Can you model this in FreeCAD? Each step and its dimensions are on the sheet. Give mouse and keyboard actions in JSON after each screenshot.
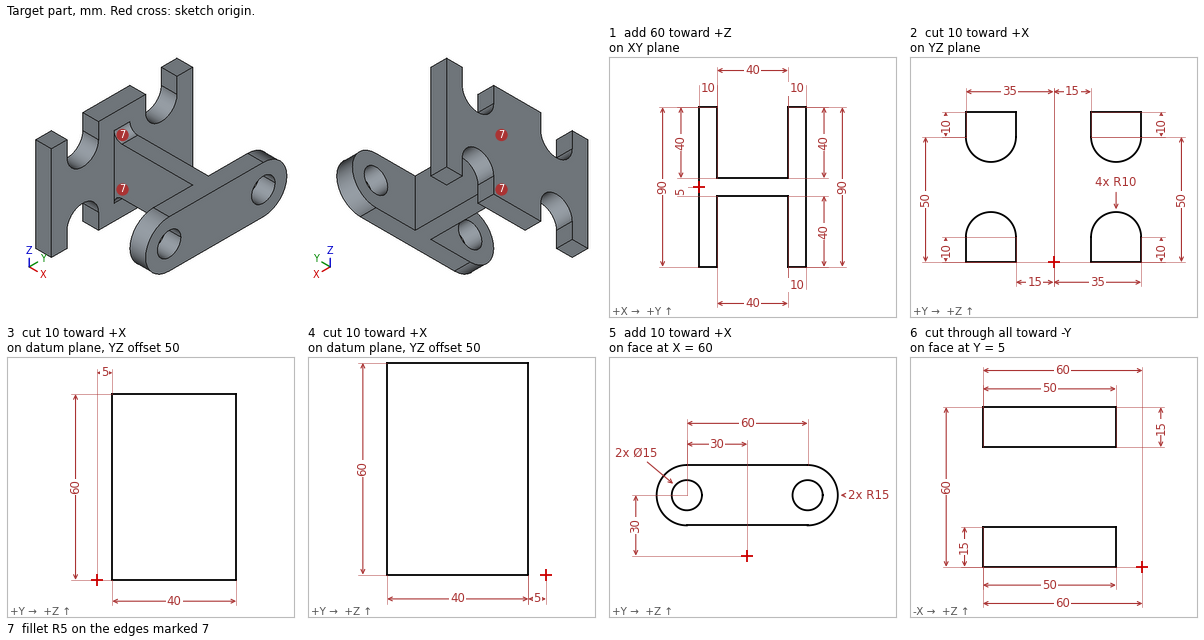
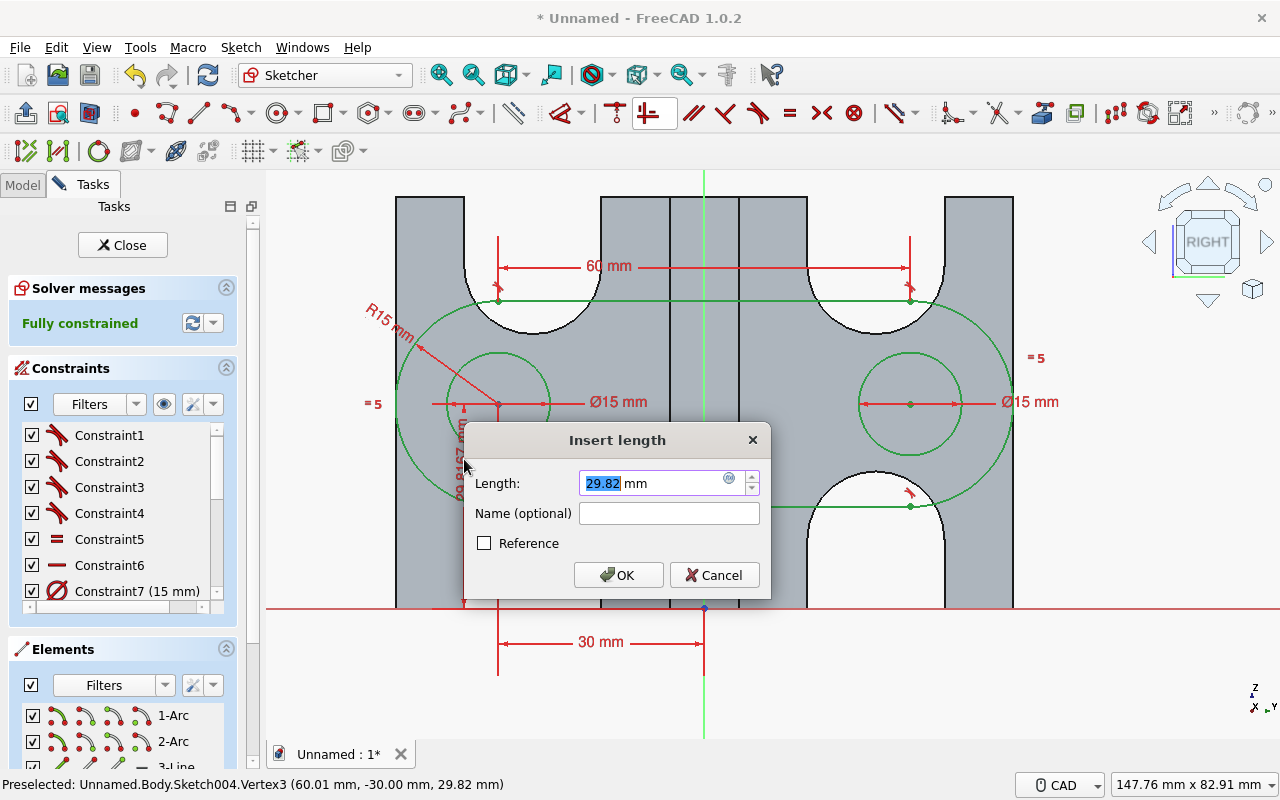
{"action": "type", "text": "30"}
{"action": "key", "text": "Return"}
{"action": "key", "text": "Escape"}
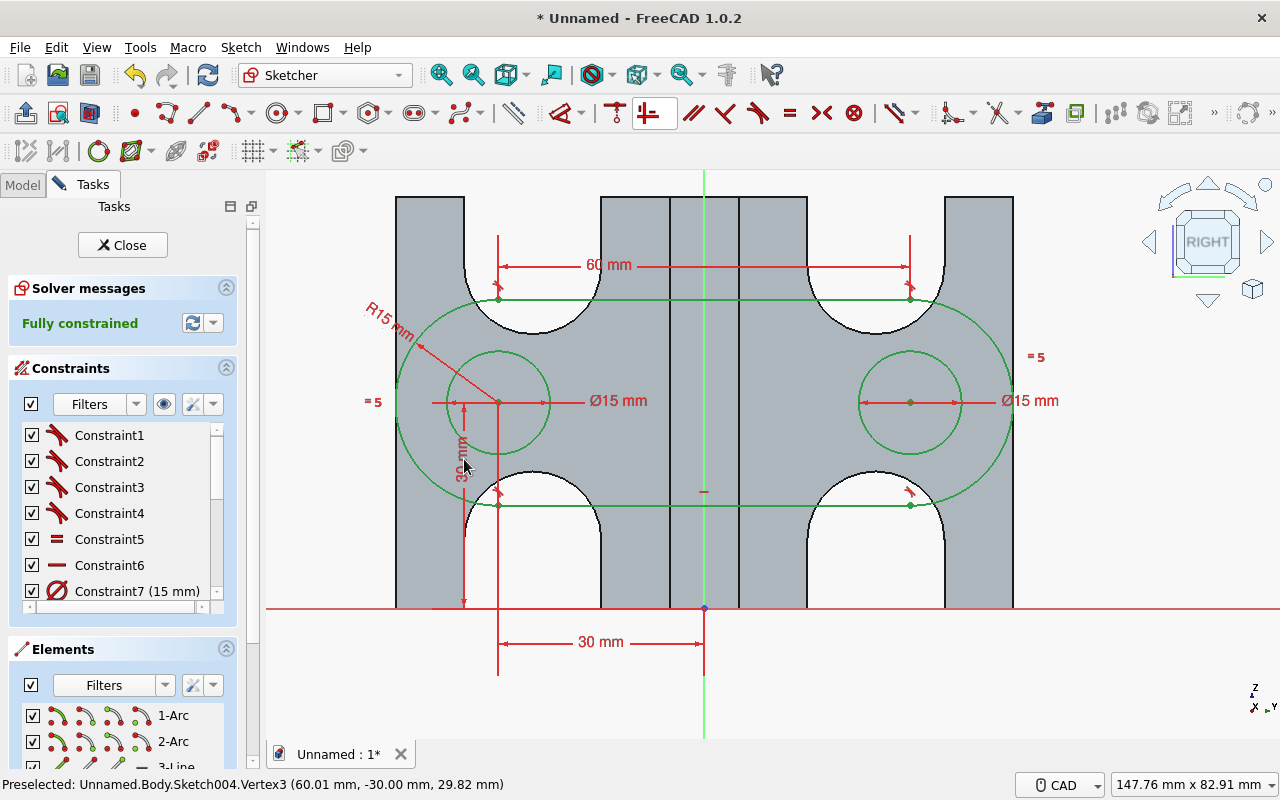
{"action": "left_click", "coordinate": [123, 245]}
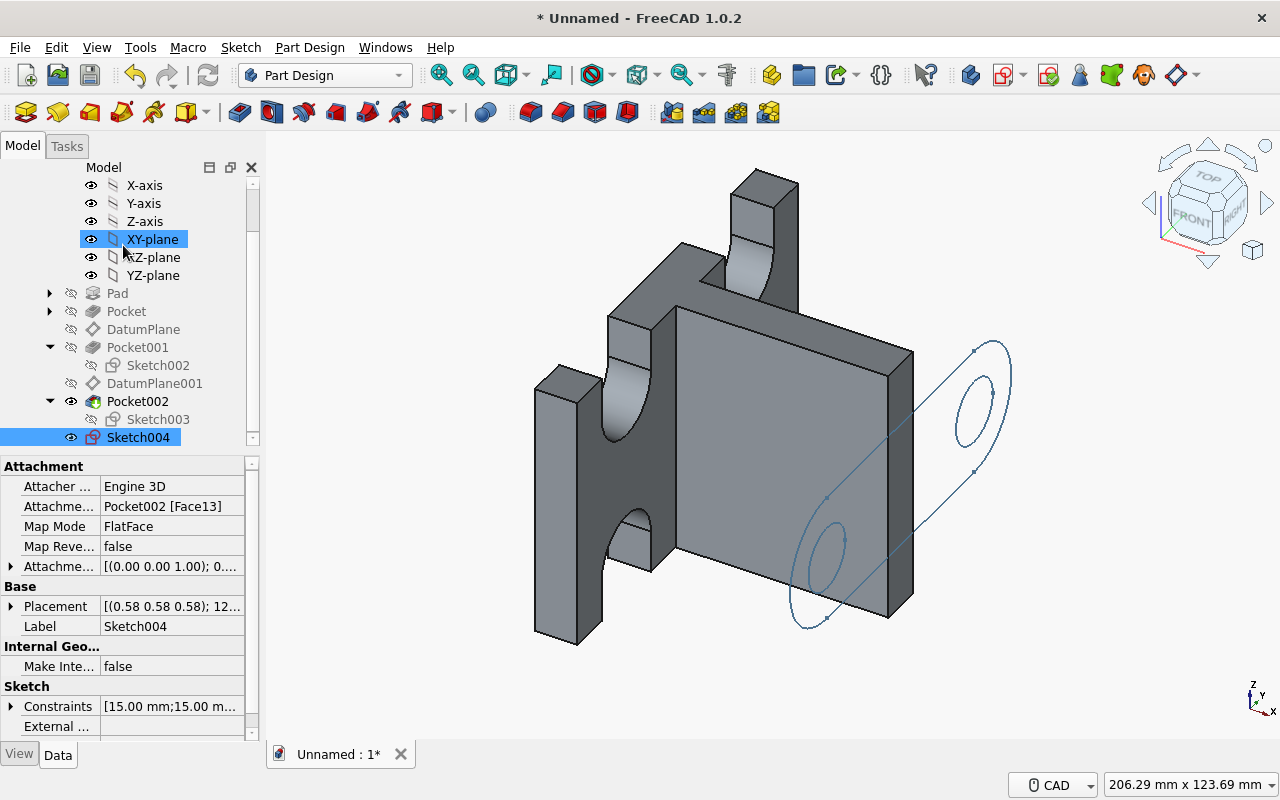
{"action": "left_click", "coordinate": [26, 112]}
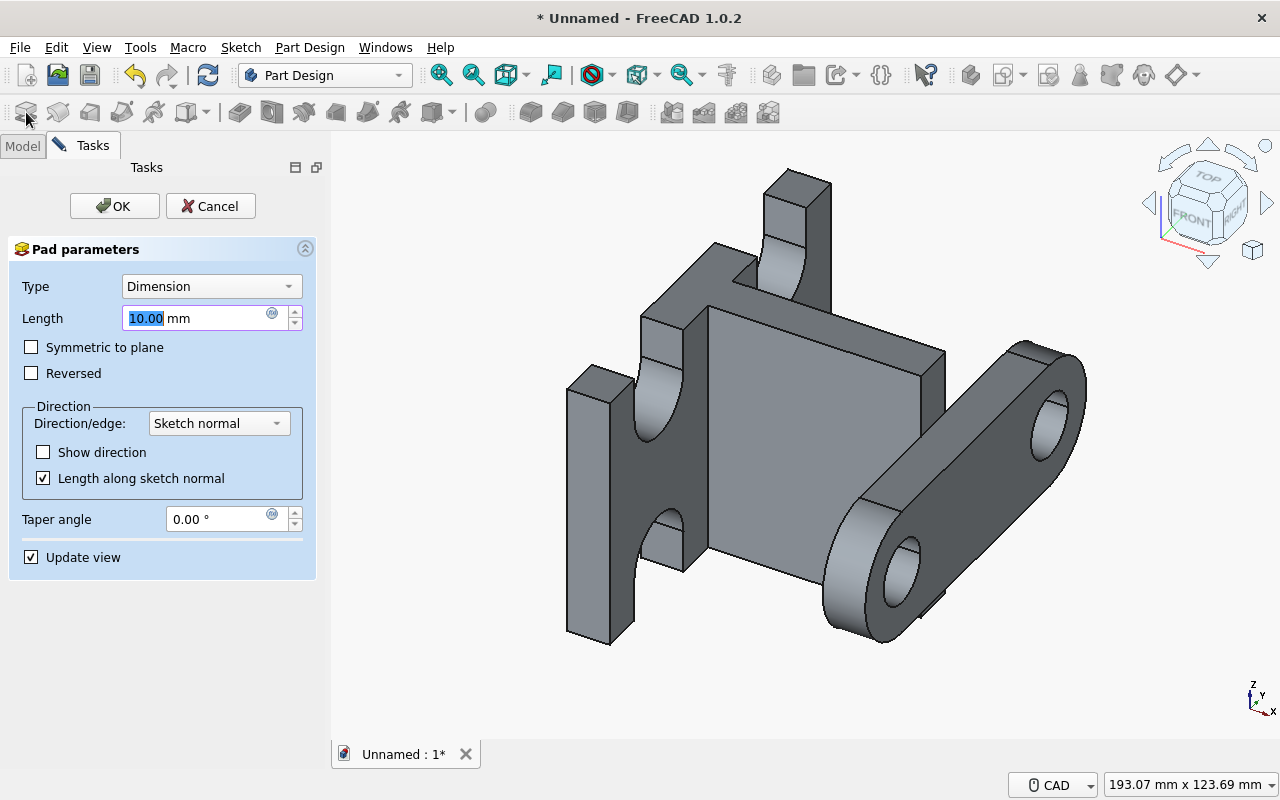
{"action": "type", "text": "10"}
{"action": "key", "text": "Tab"}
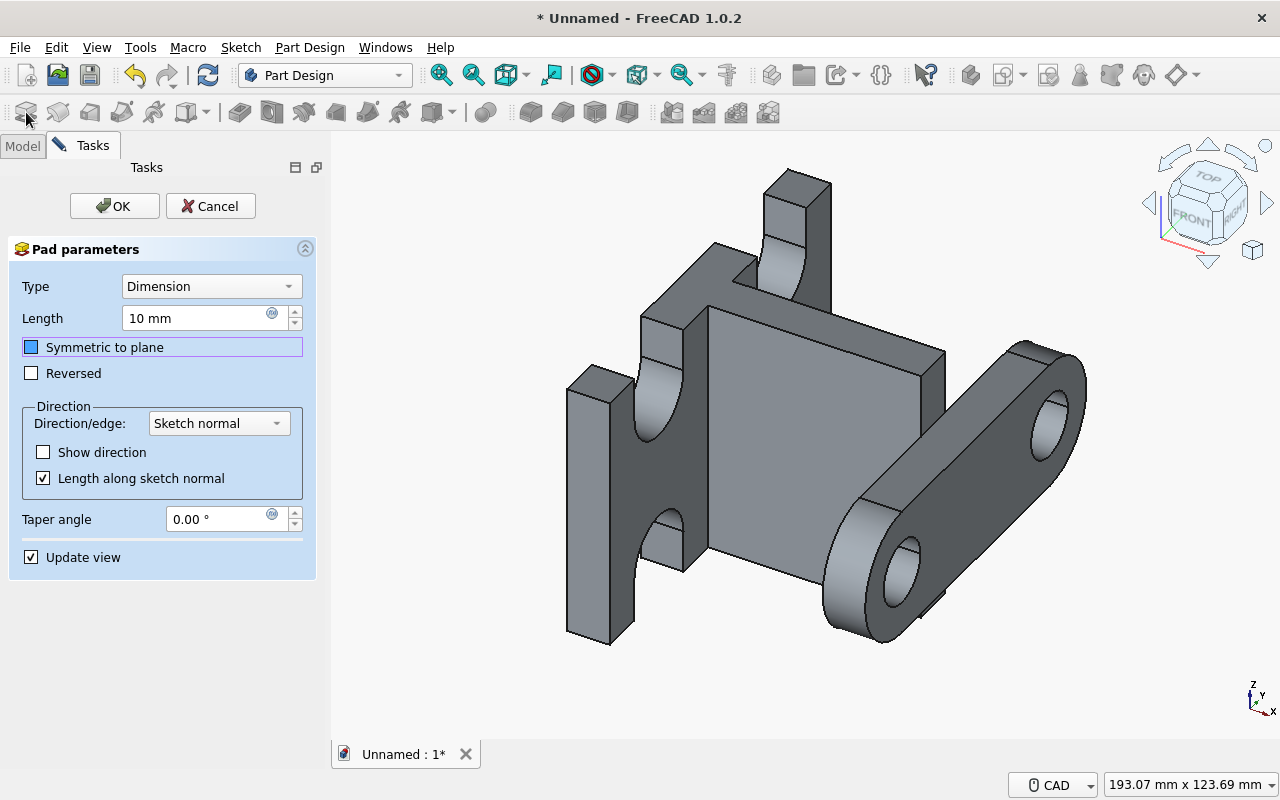
{"action": "left_click", "coordinate": [115, 206]}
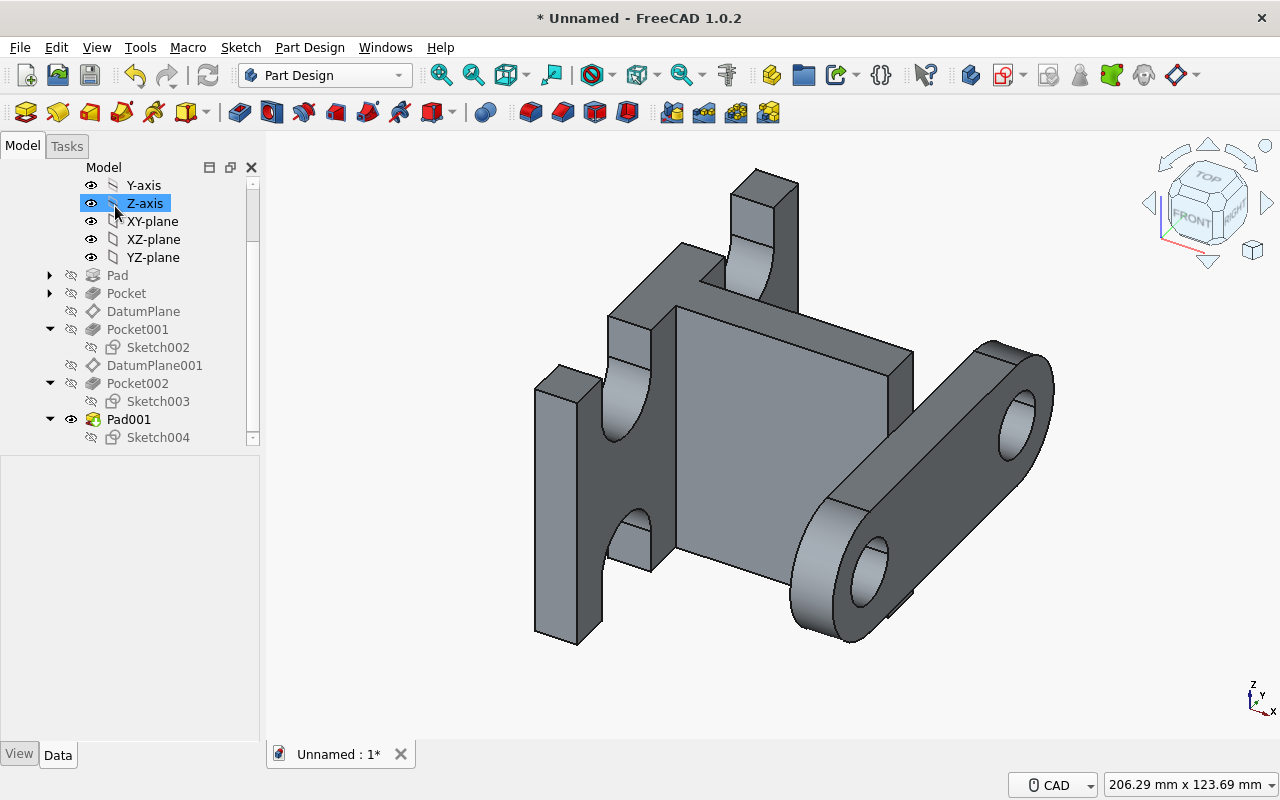
{"action": "key", "text": "4"}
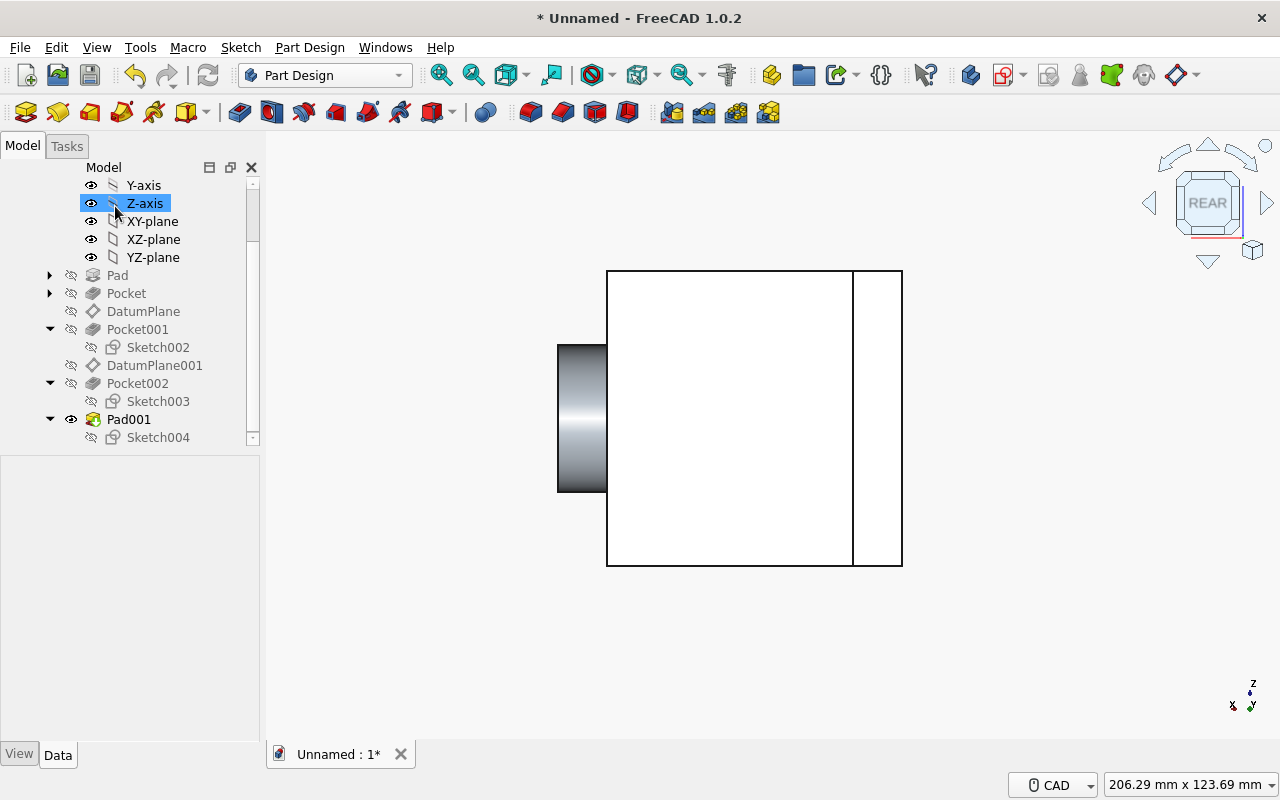
{"action": "left_click", "coordinate": [730, 417]}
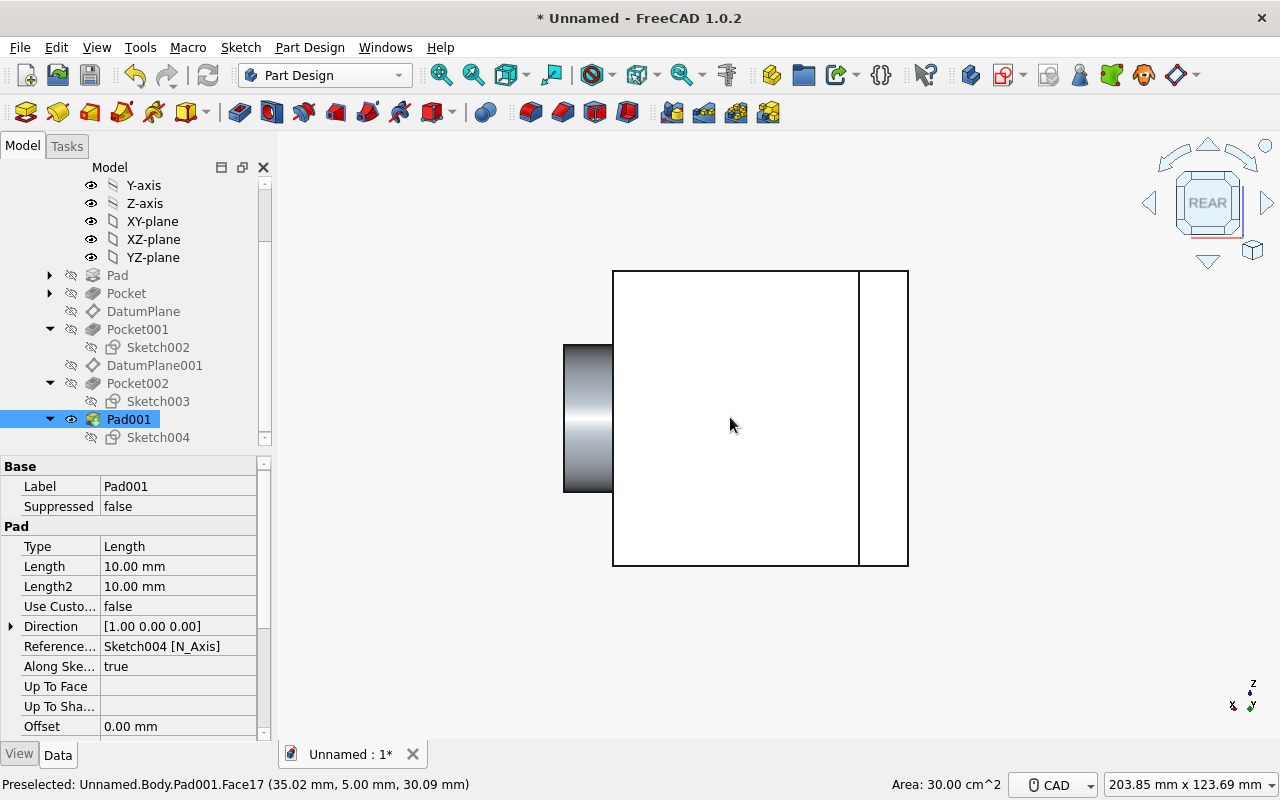
{"action": "left_click", "coordinate": [1004, 76]}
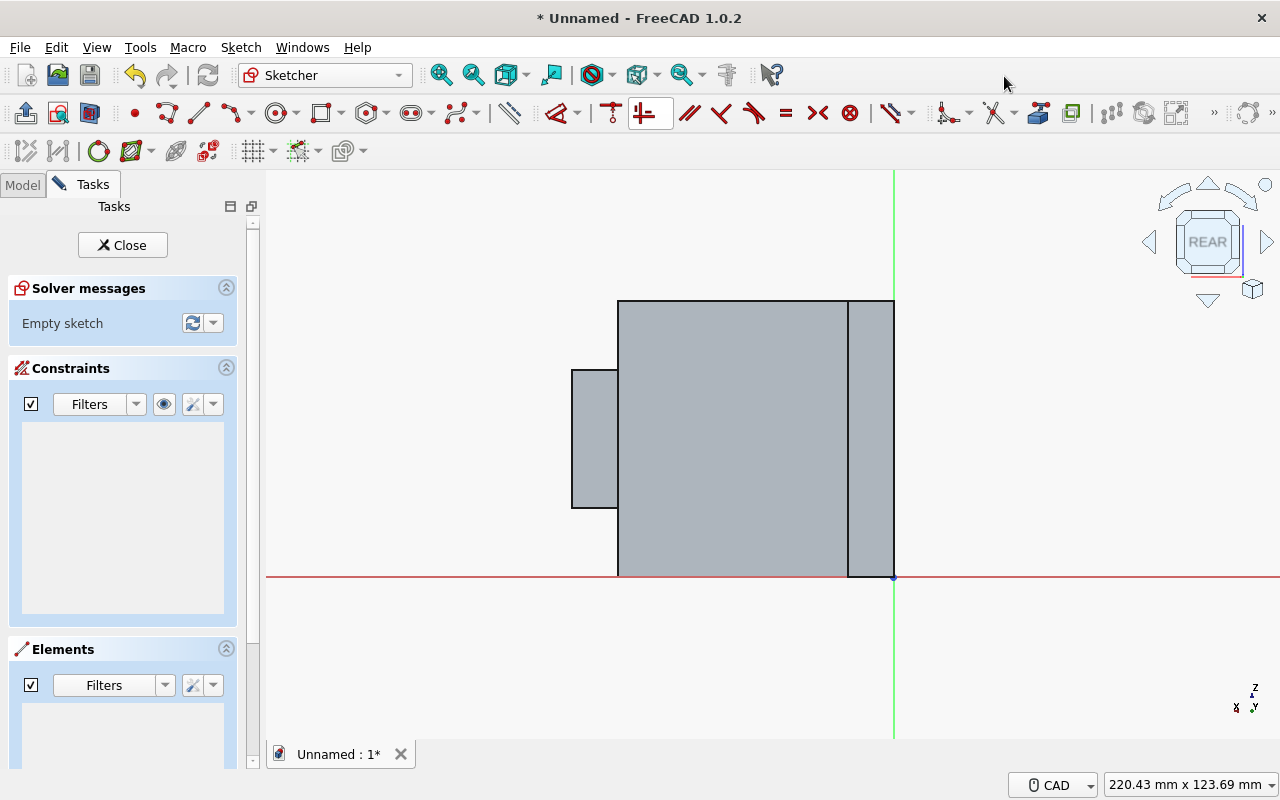
{"action": "left_click", "coordinate": [90, 114]}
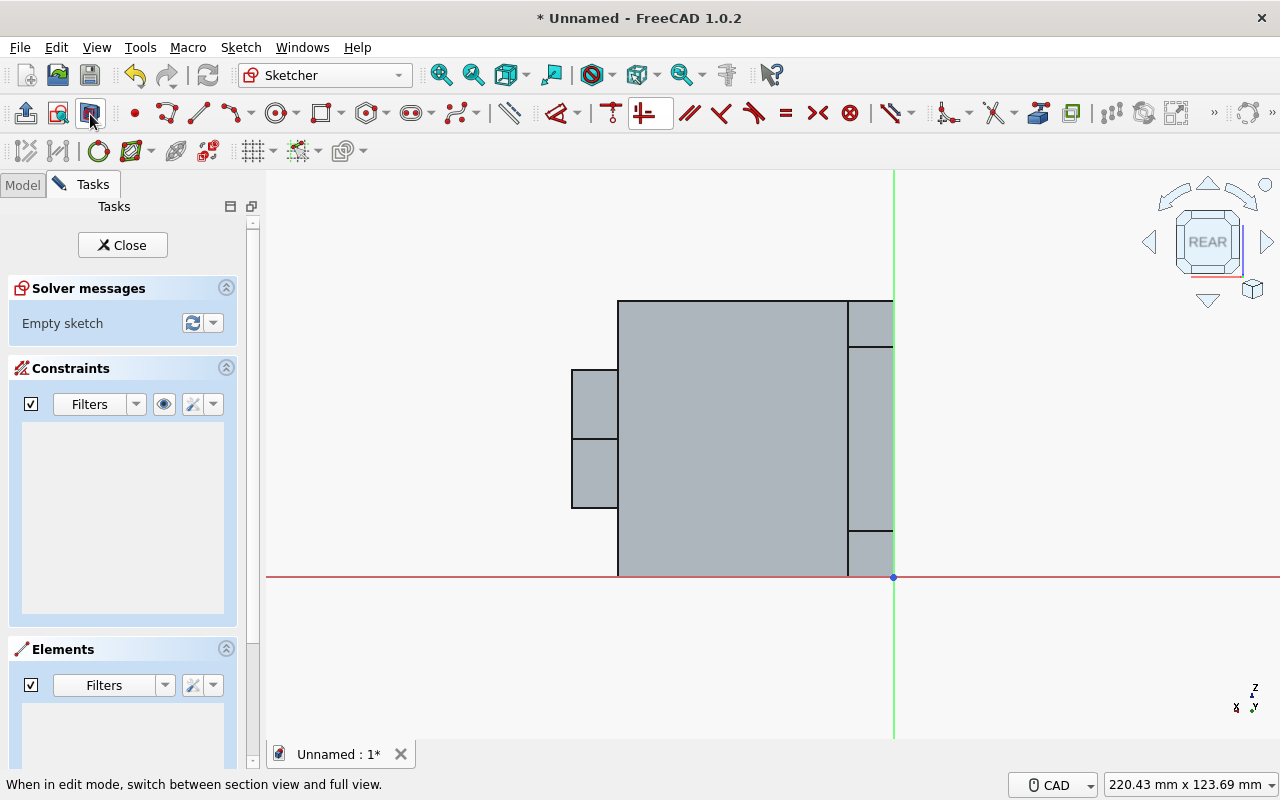
{"action": "left_click", "coordinate": [322, 114]}